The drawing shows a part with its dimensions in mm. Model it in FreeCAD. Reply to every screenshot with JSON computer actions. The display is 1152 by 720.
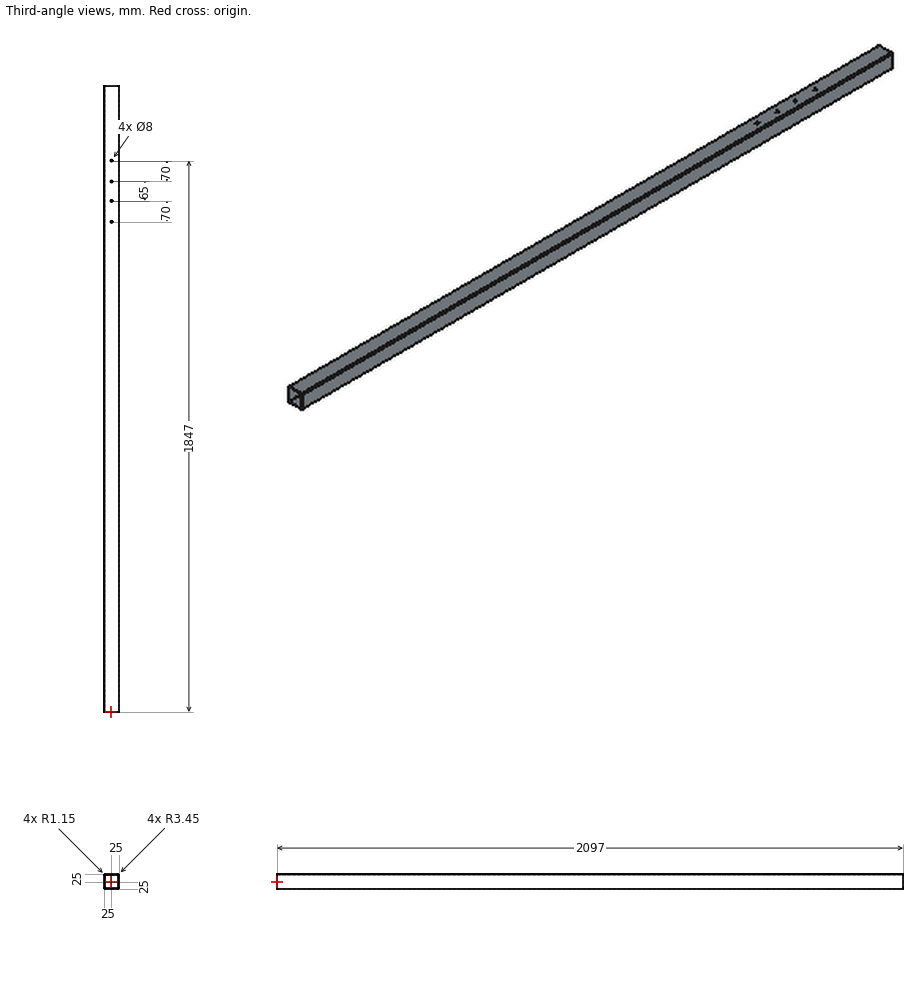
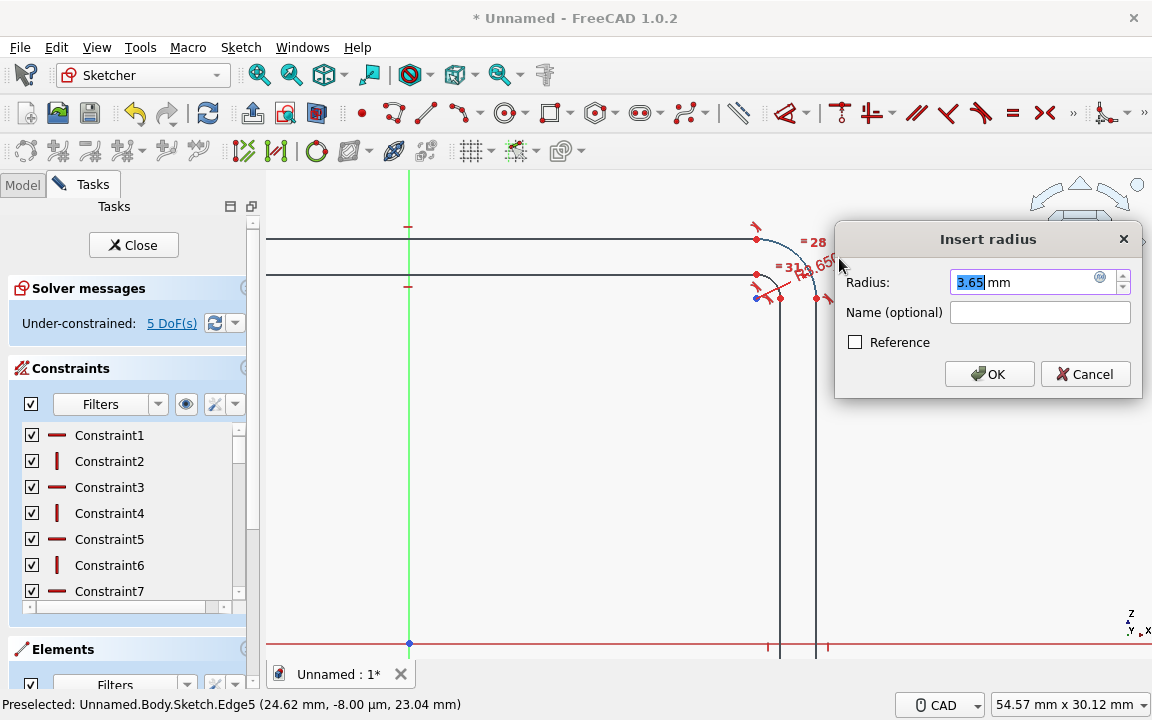
{"action": "type", "text": "3.45"}
{"action": "key", "text": "Return"}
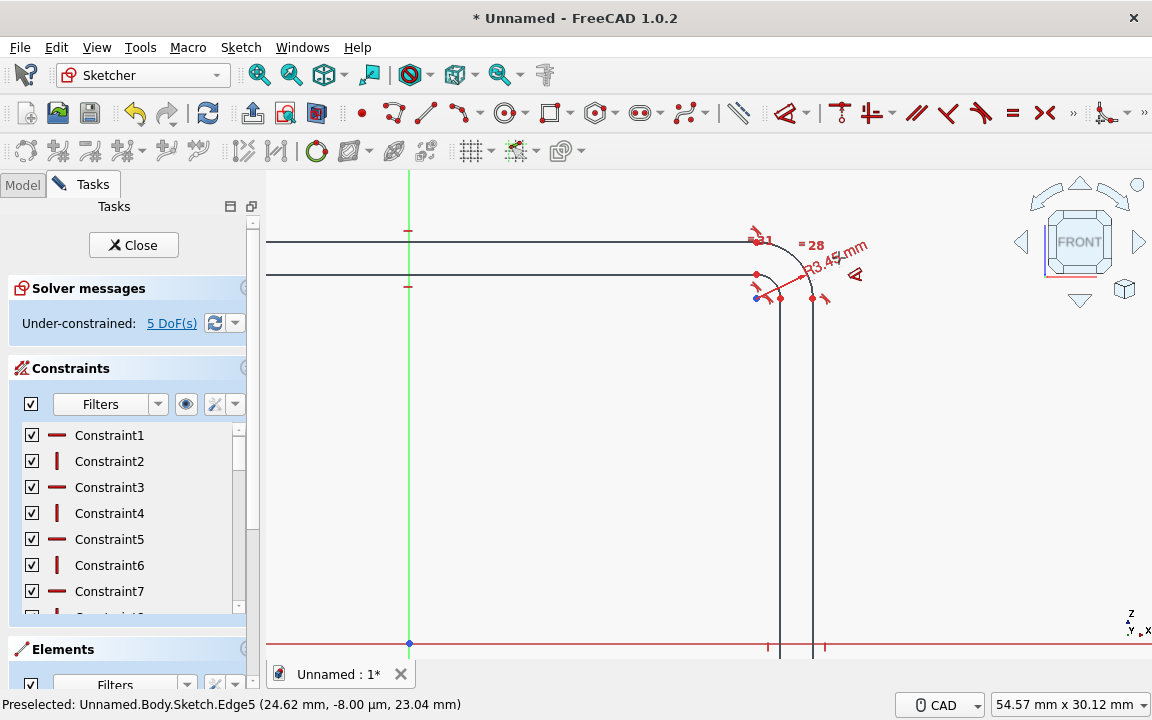
{"action": "scroll", "coordinate": [775, 281], "scroll_direction": "down", "scroll_amount": 5}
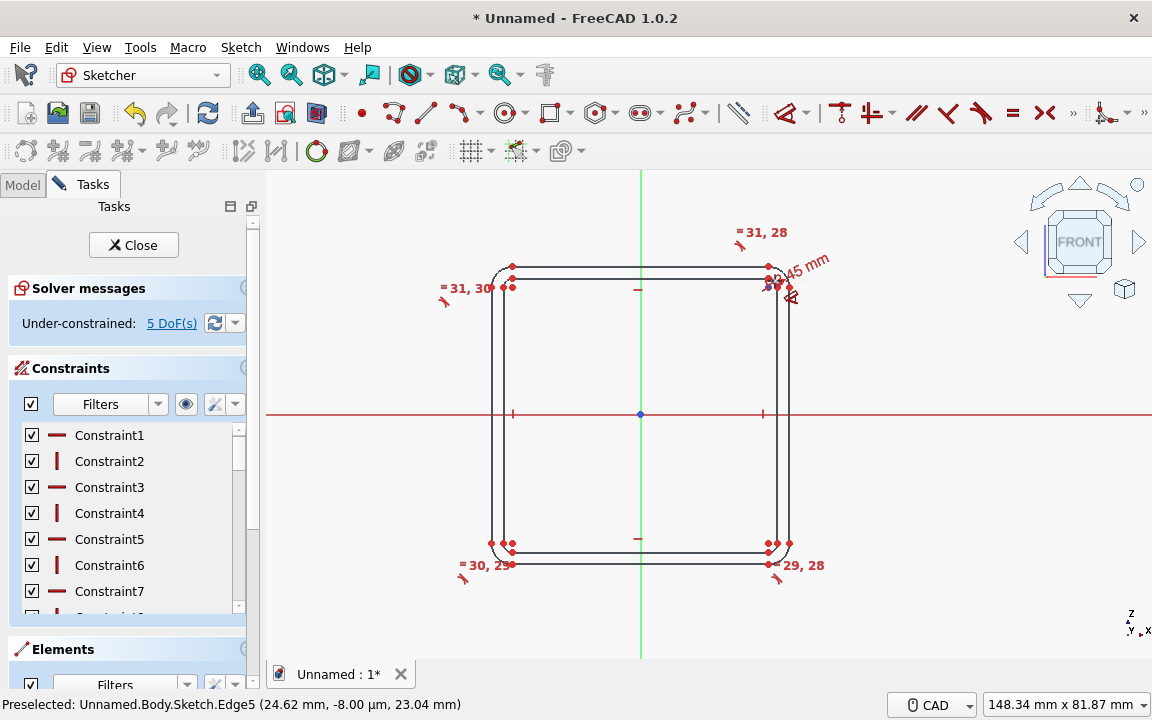
{"action": "scroll", "coordinate": [508, 280], "scroll_direction": "up", "scroll_amount": 9}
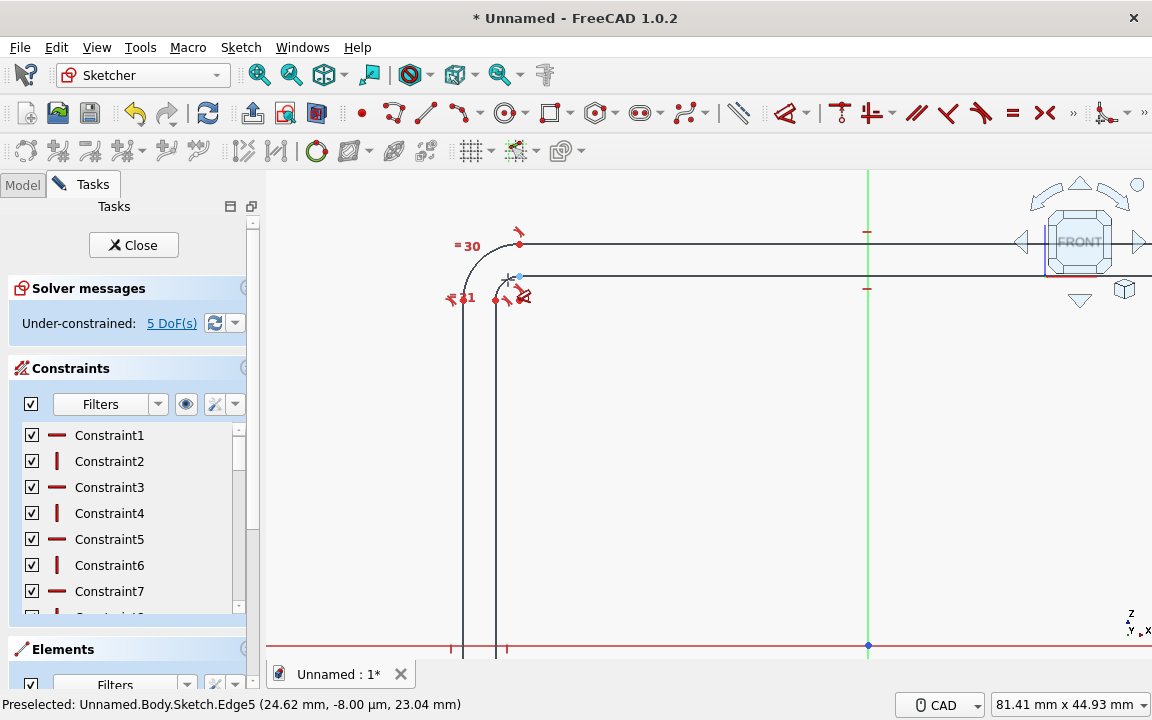
{"action": "left_click", "coordinate": [509, 278]}
{"action": "left_click", "coordinate": [494, 250]}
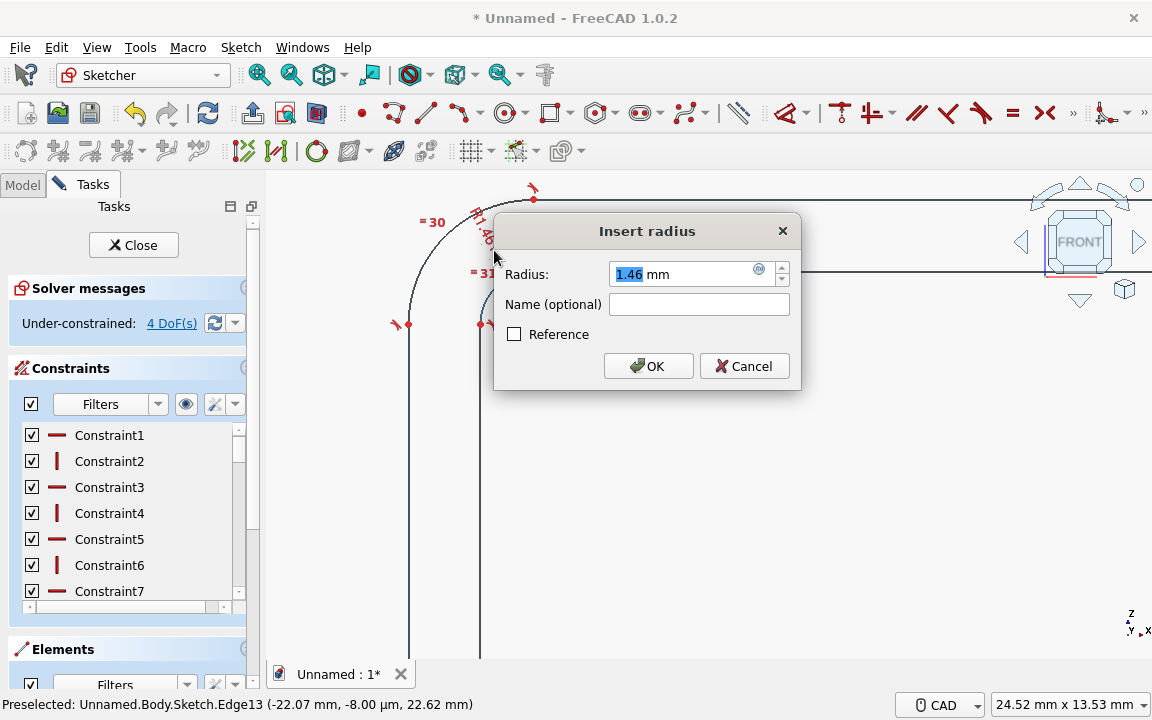
{"action": "type", "text": "1.15"}
{"action": "key", "text": "Return"}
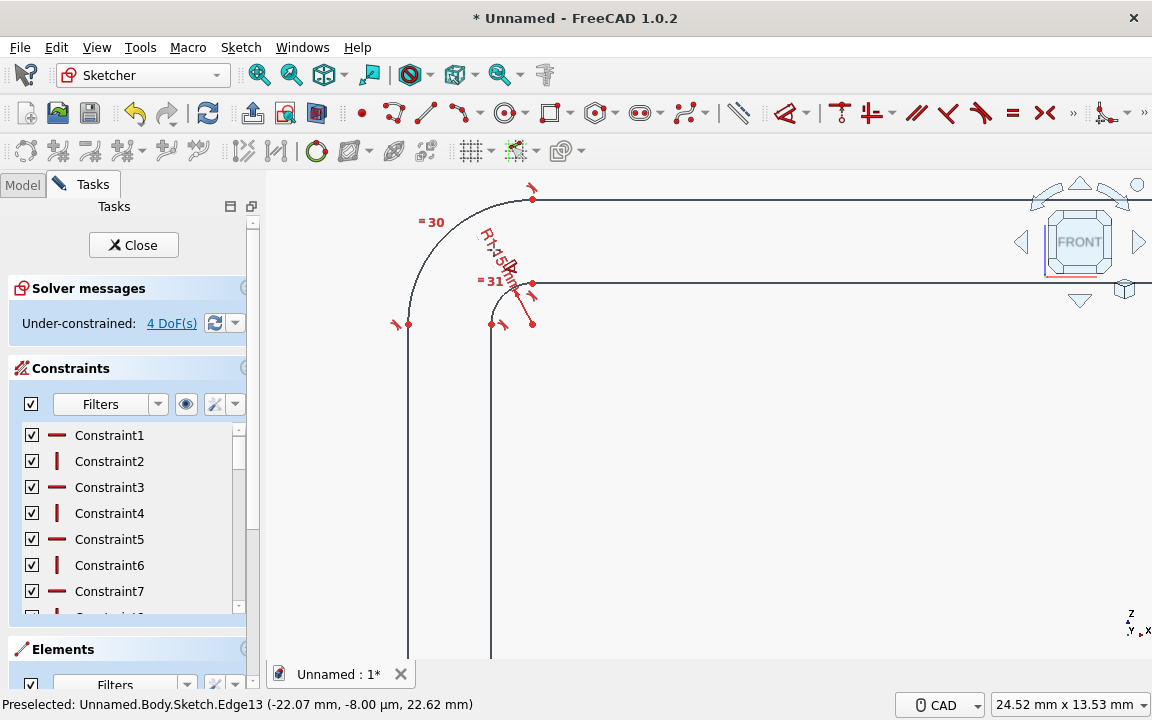
{"action": "scroll", "coordinate": [508, 280], "scroll_direction": "down", "scroll_amount": 9}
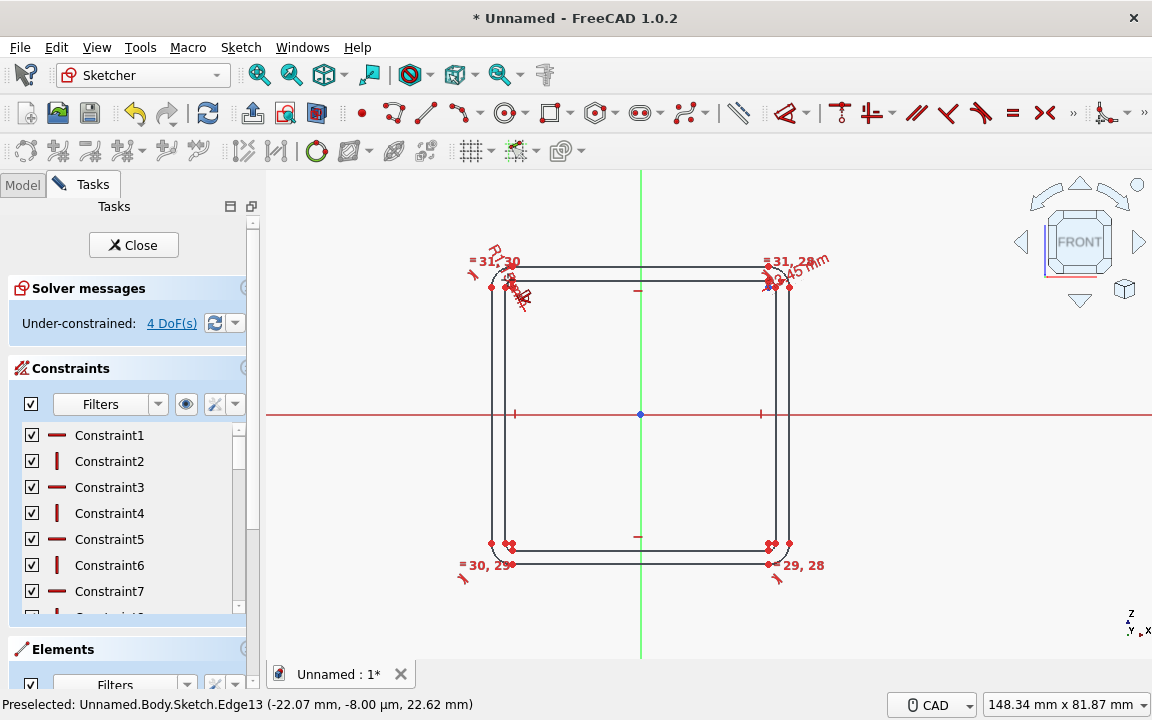
{"action": "left_click", "coordinate": [512, 267]}
{"action": "left_click", "coordinate": [478, 341]}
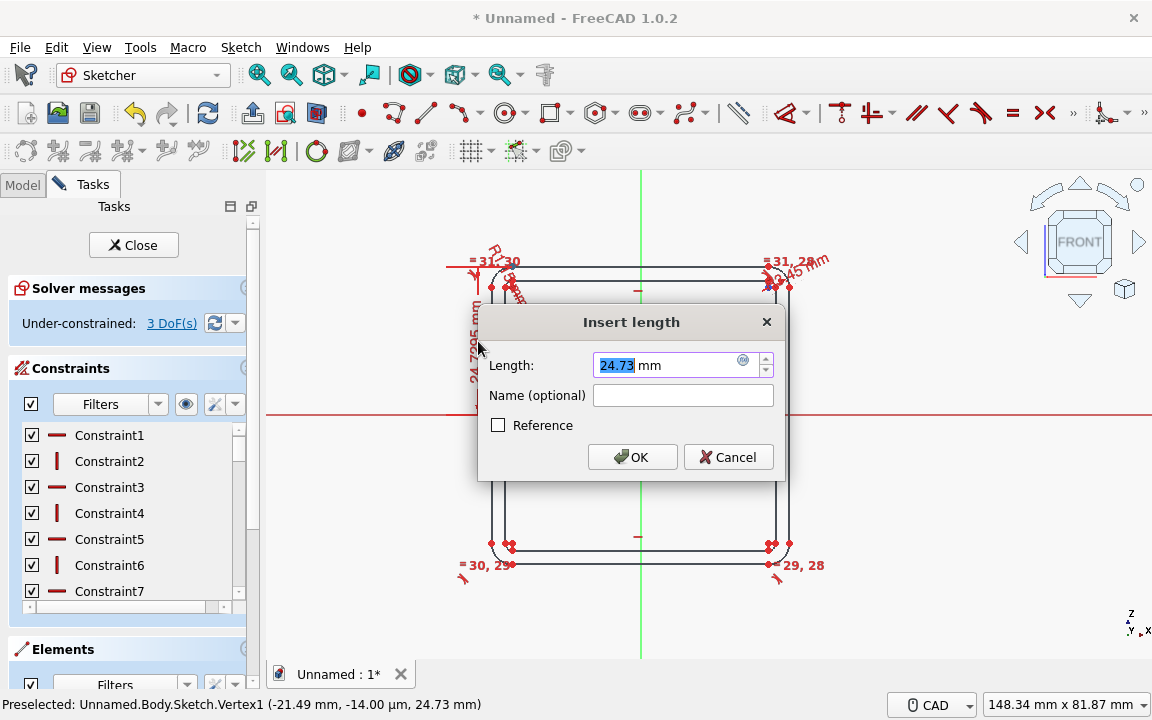
{"action": "type", "text": "25"}
{"action": "key", "text": "Return"}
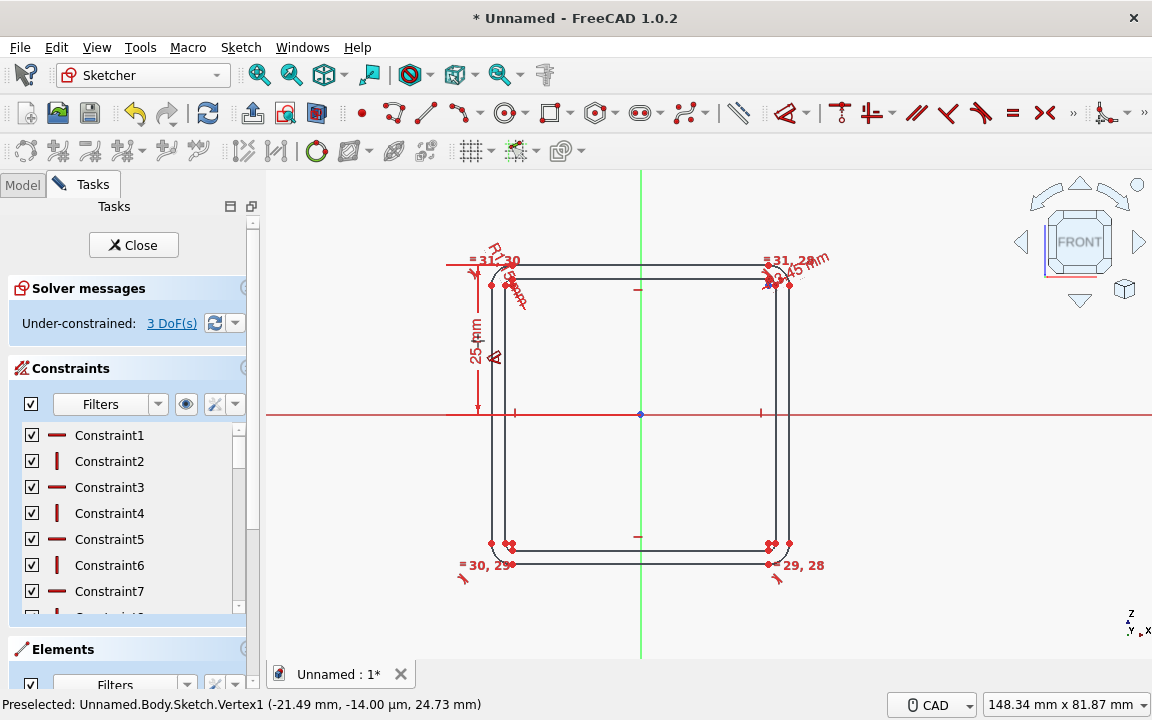
{"action": "left_click", "coordinate": [789, 286]}
{"action": "left_click", "coordinate": [715, 252]}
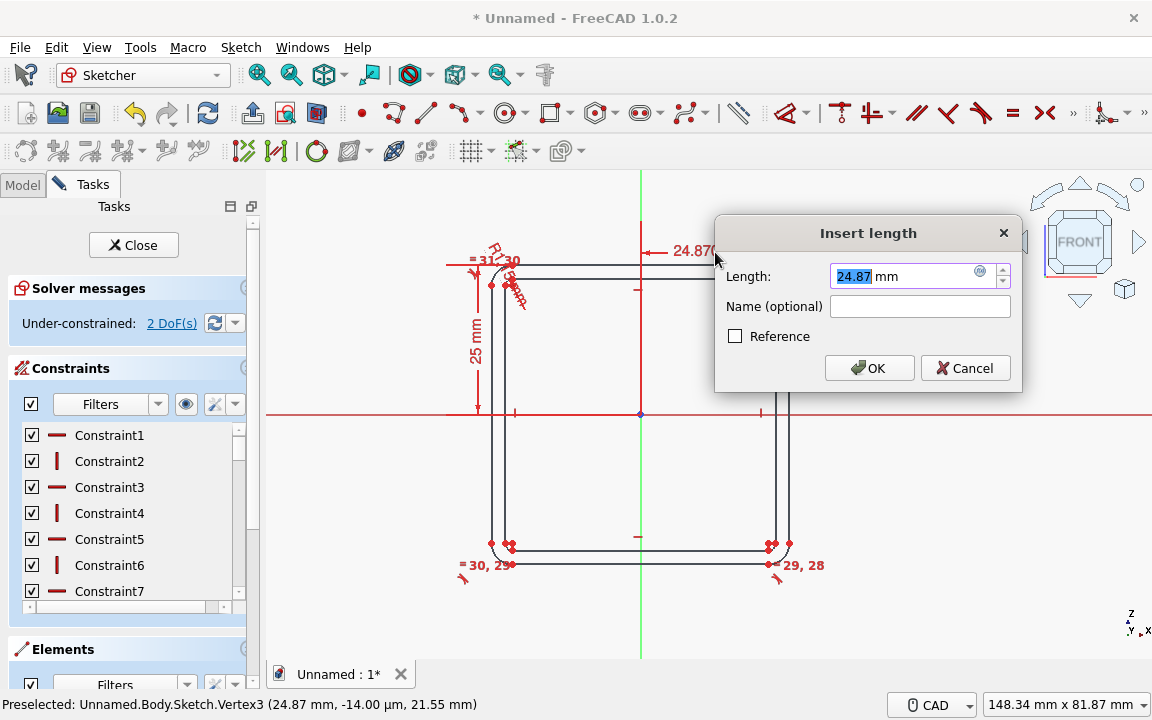
{"action": "type", "text": "25"}
{"action": "key", "text": "Return"}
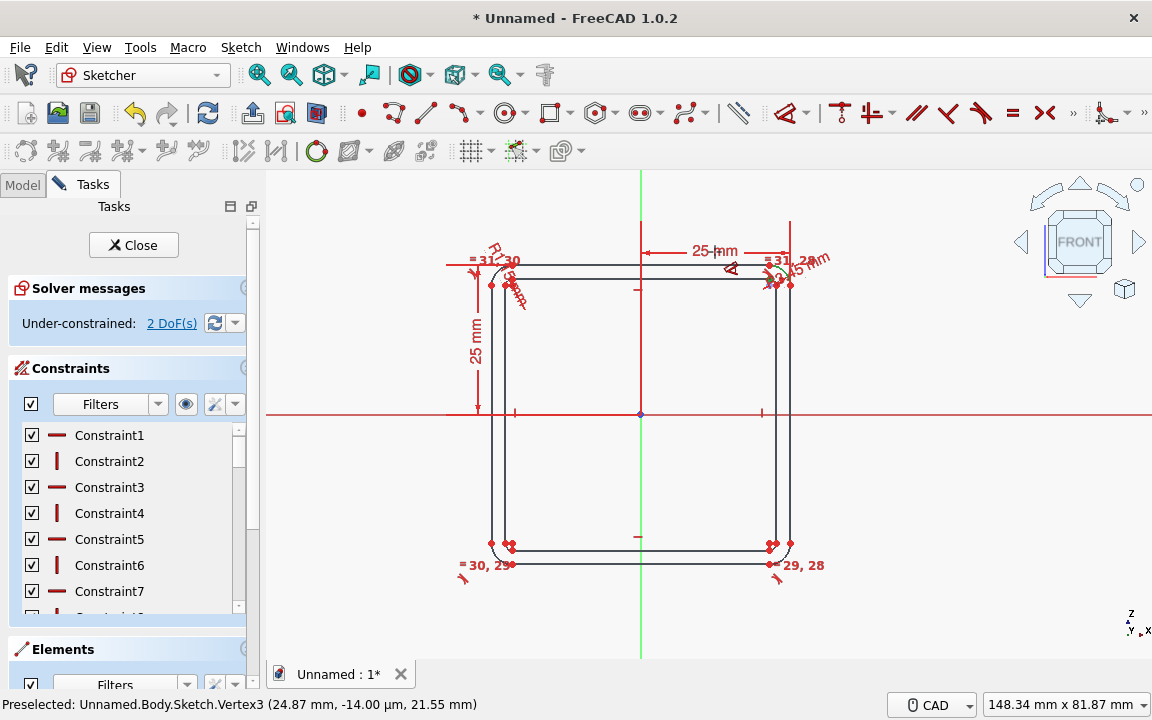
{"action": "left_click", "coordinate": [769, 564]}
{"action": "left_click", "coordinate": [803, 490]}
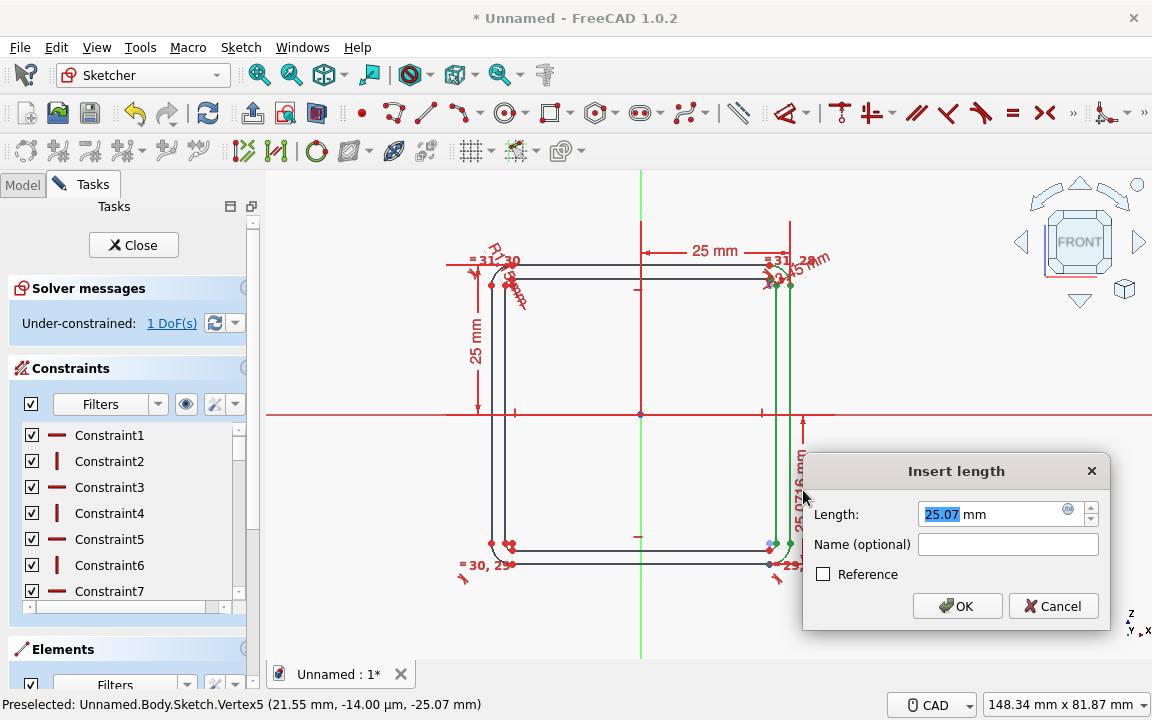
{"action": "type", "text": "25"}
{"action": "key", "text": "Return"}